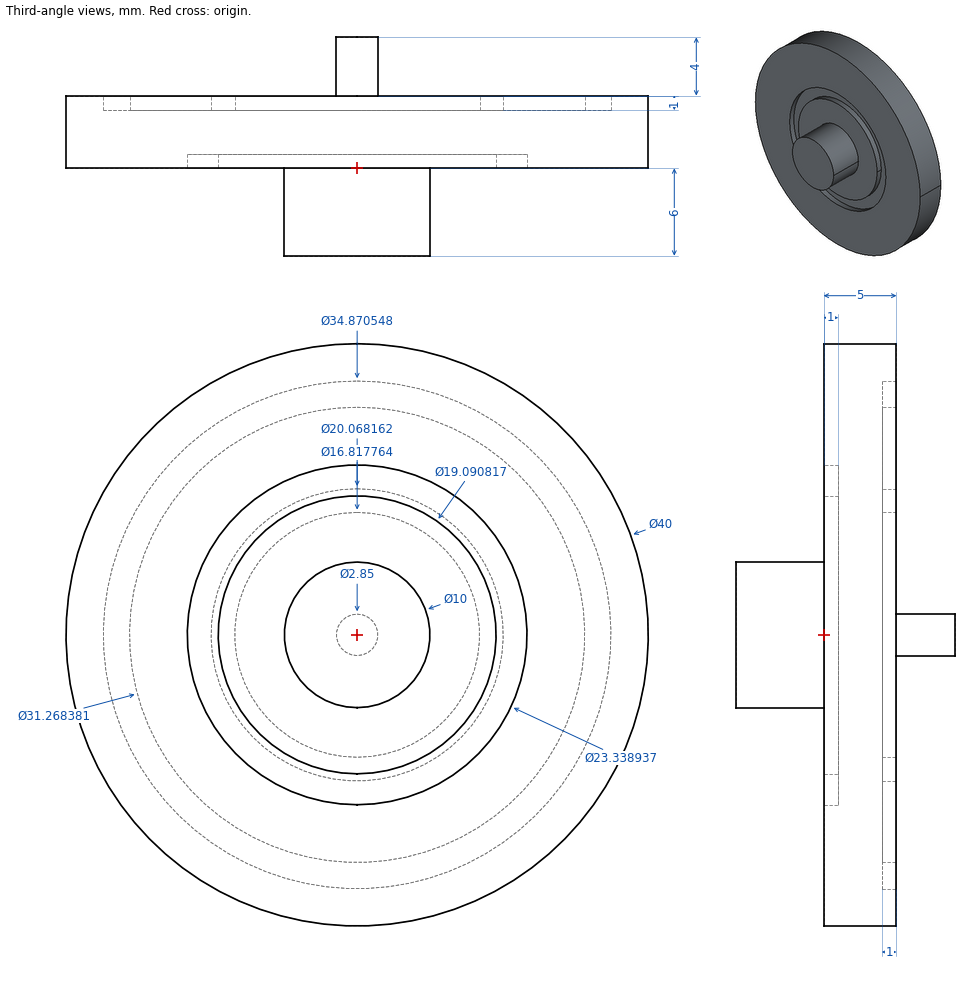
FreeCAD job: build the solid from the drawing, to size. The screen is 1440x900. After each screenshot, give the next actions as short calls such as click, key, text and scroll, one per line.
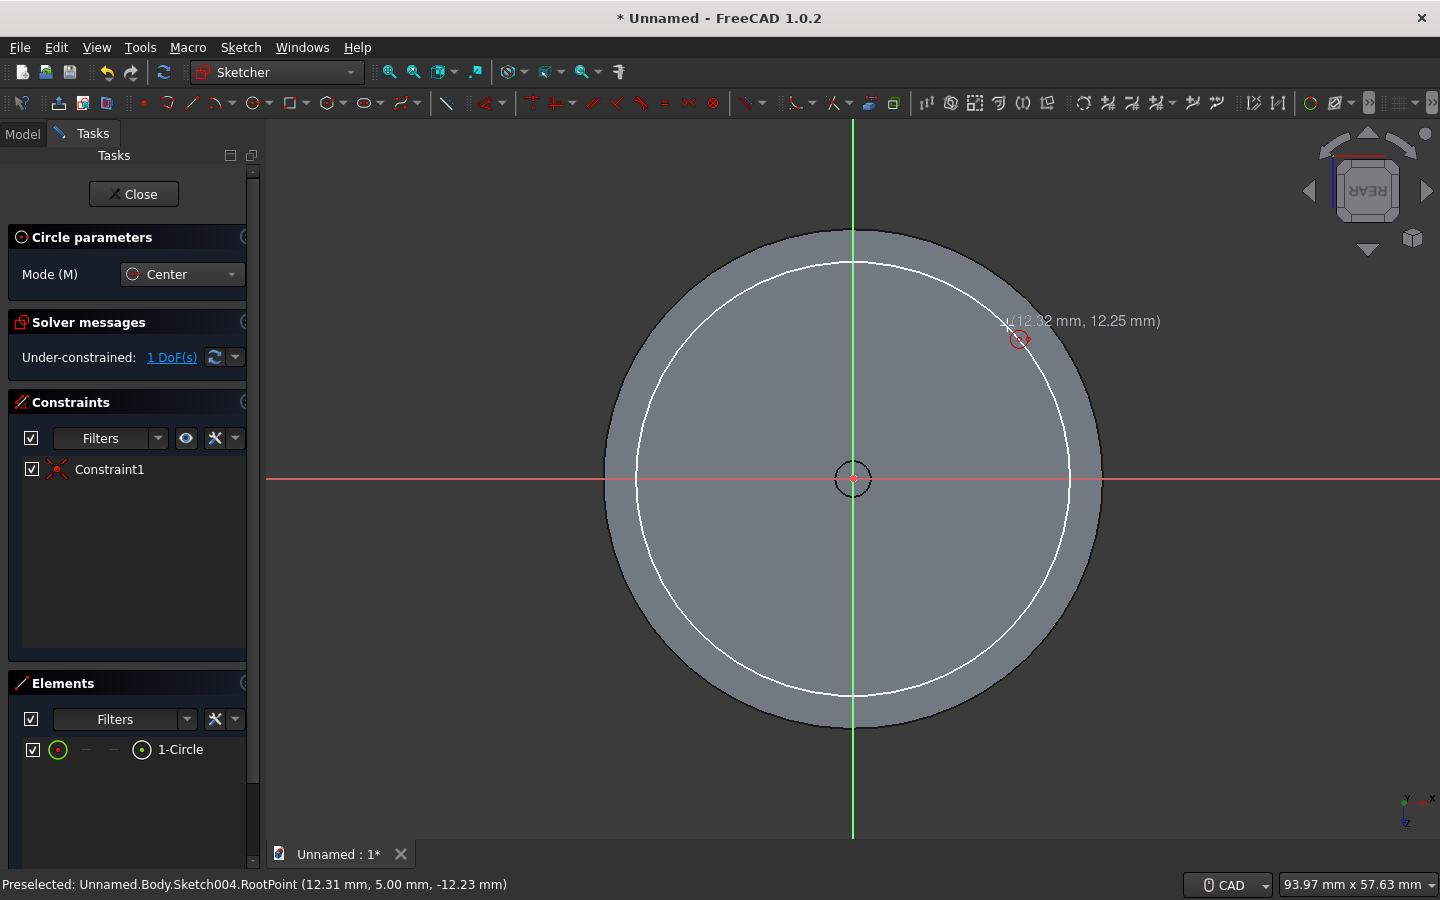
click(853, 479)
click(991, 341)
key(Escape)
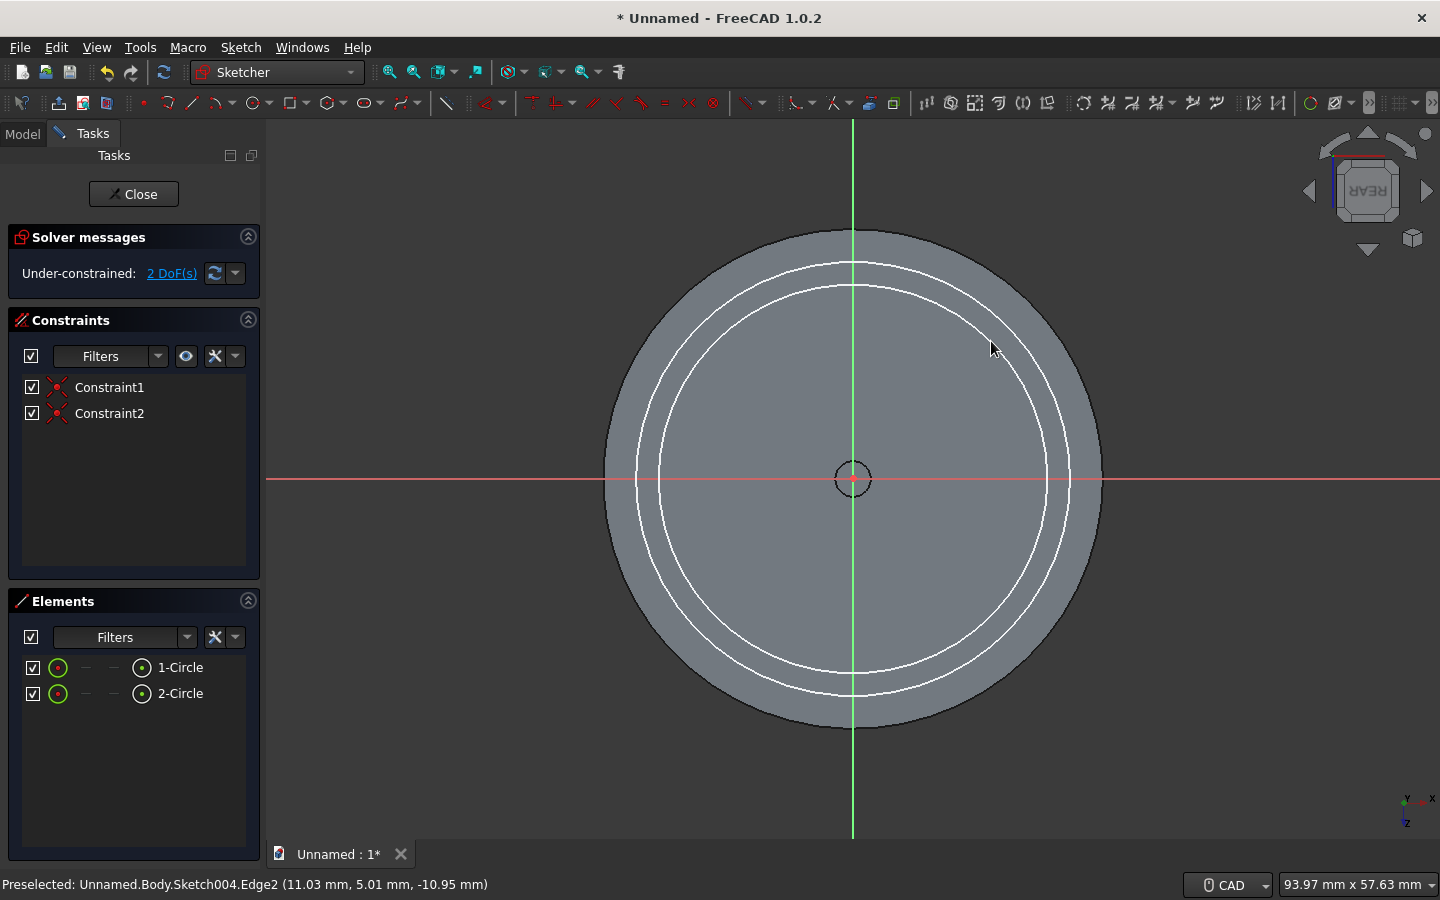
click(486, 104)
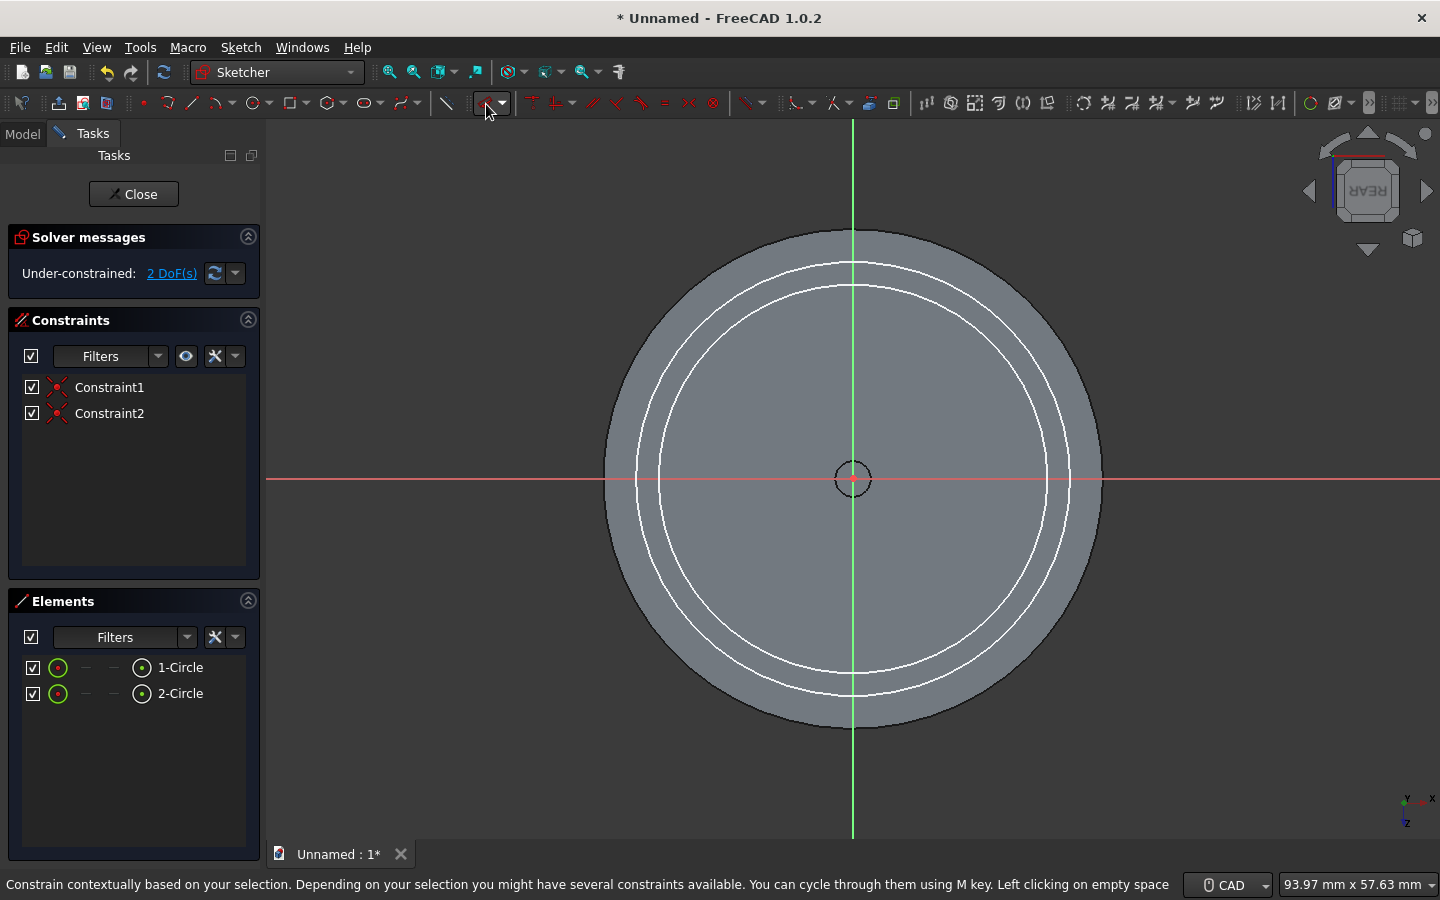
click(1006, 325)
click(1029, 302)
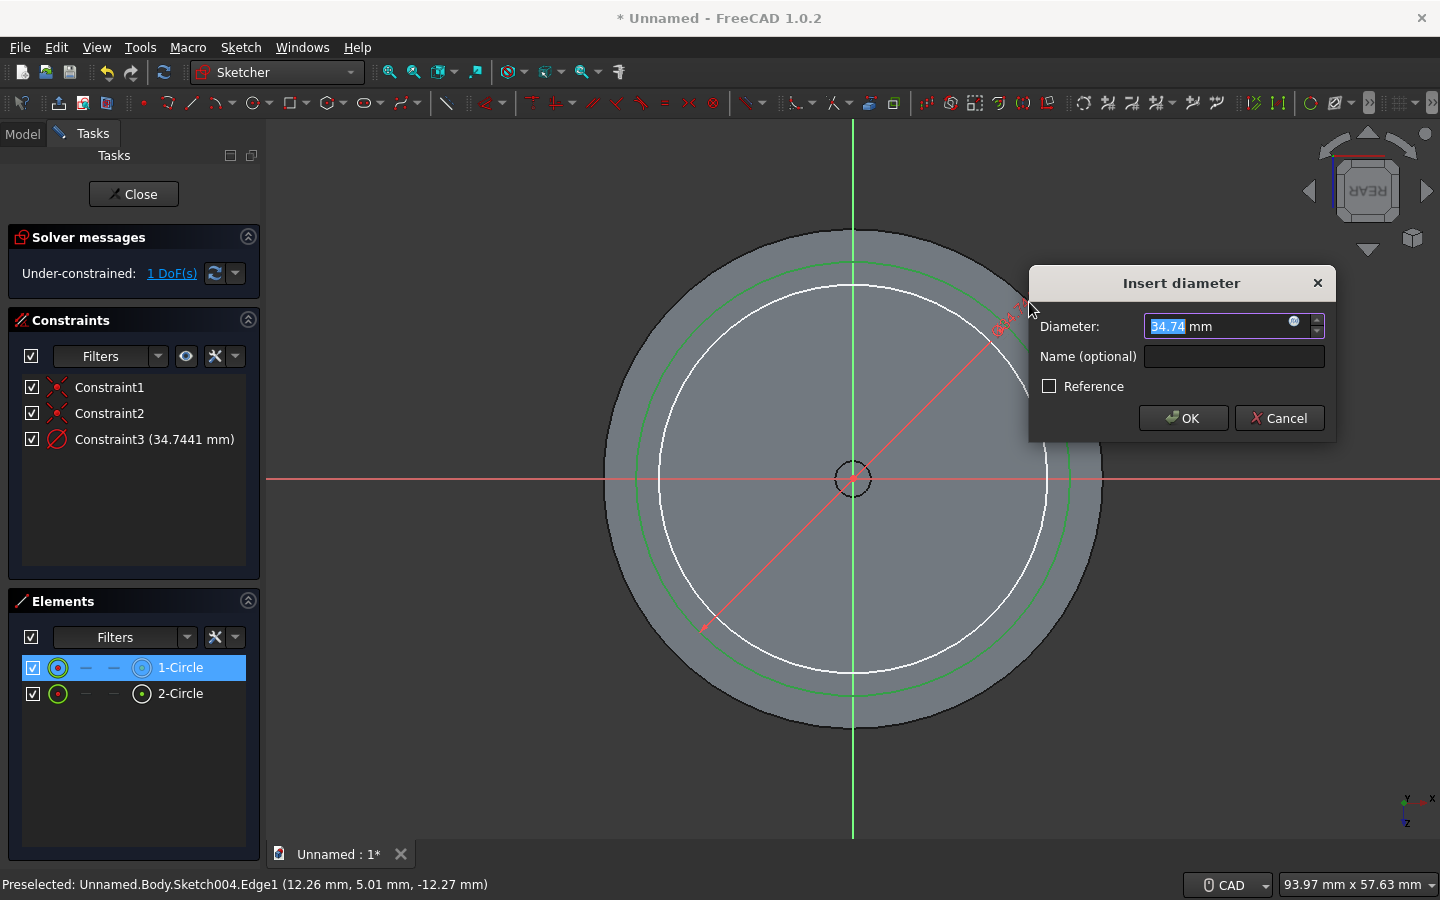
text(34.870548)
key(Return)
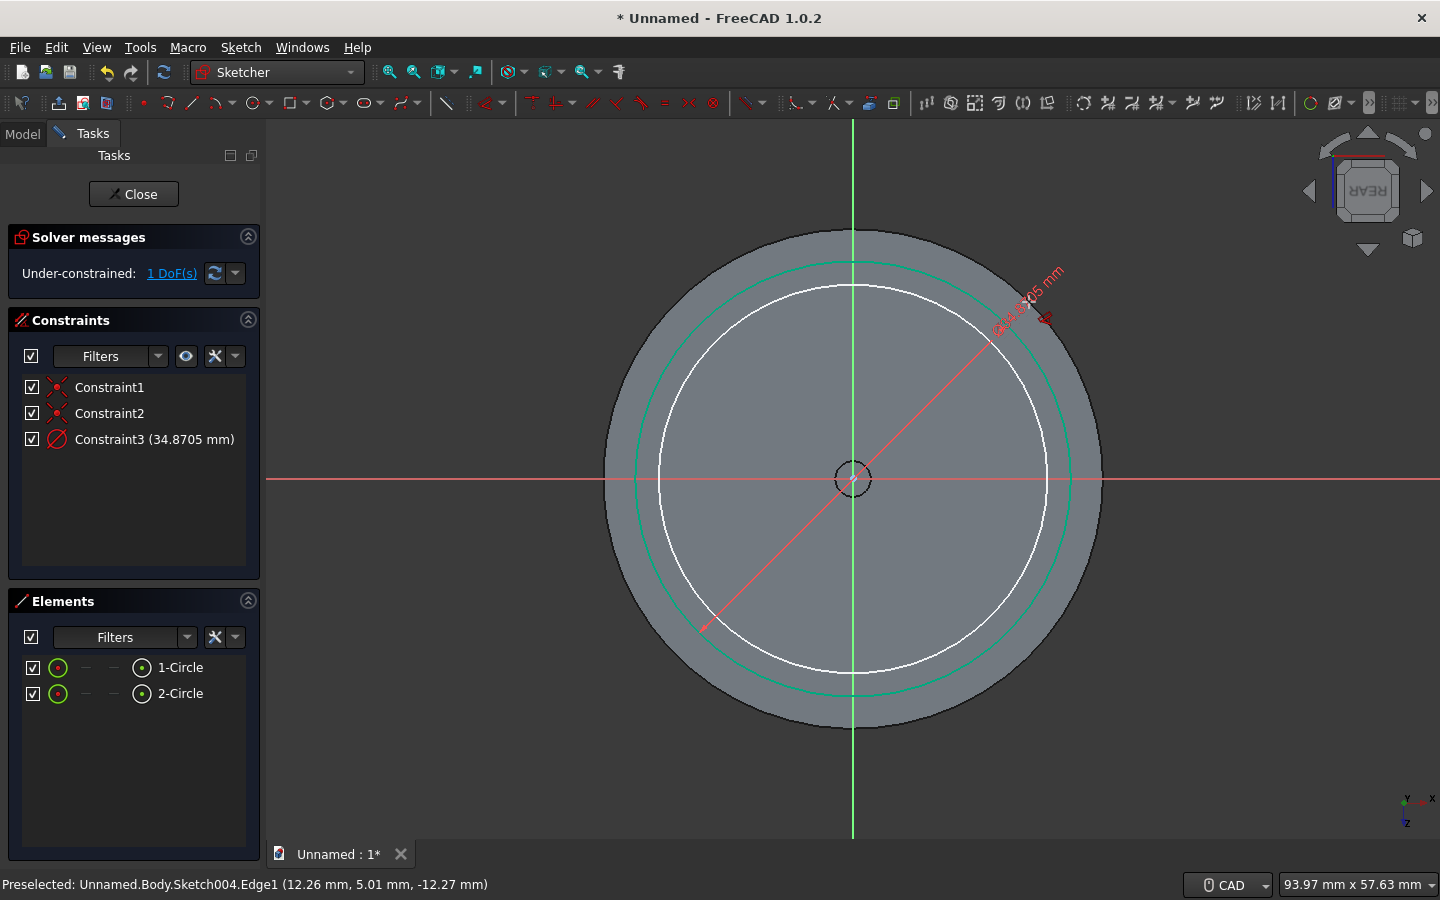
click(990, 341)
click(1092, 408)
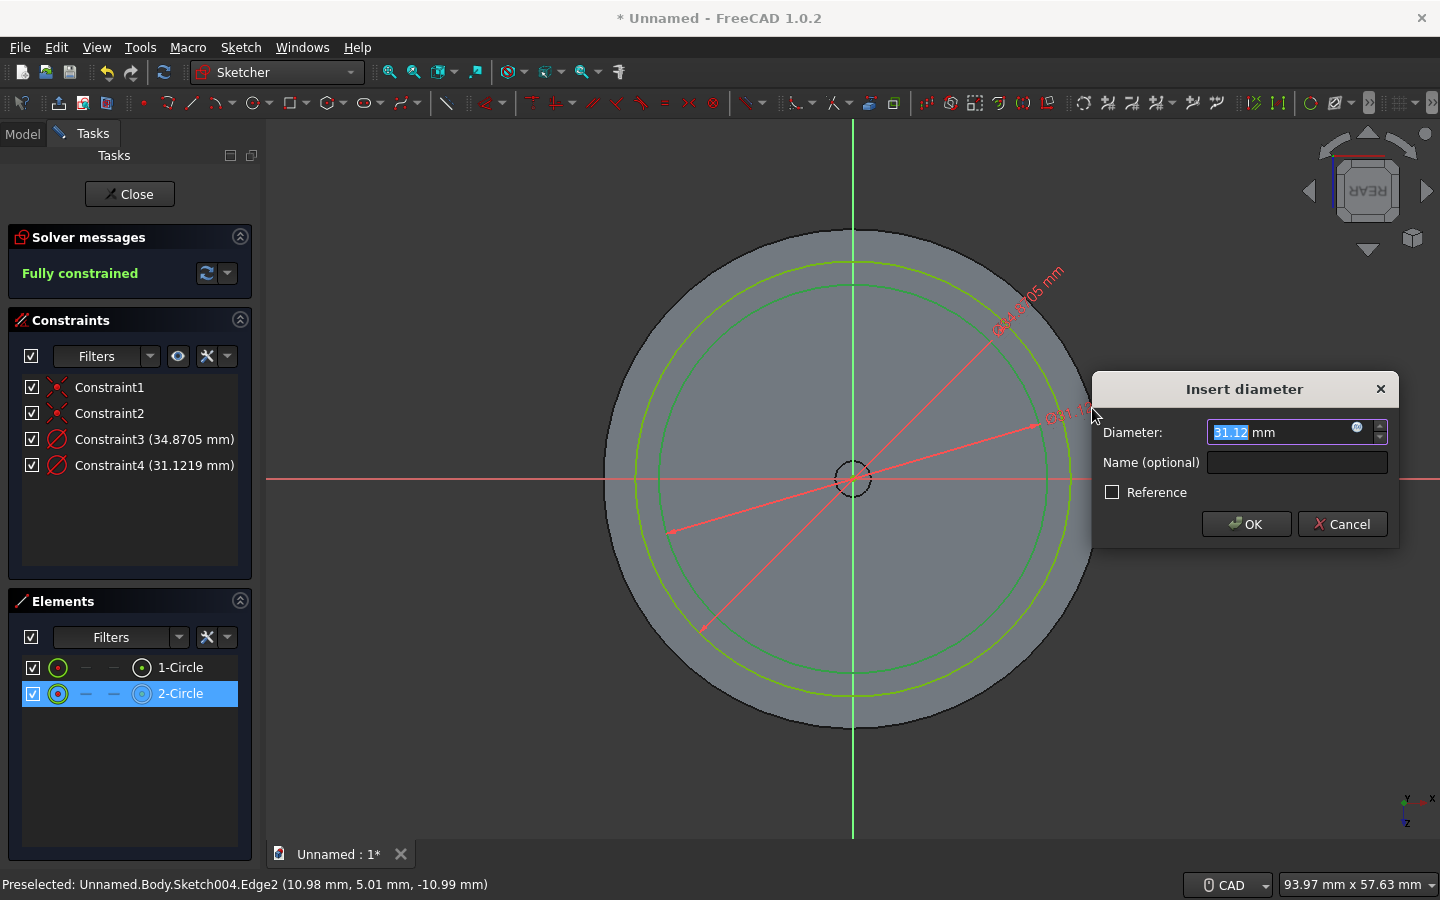
text(31.268381)
key(Return)
key(Escape)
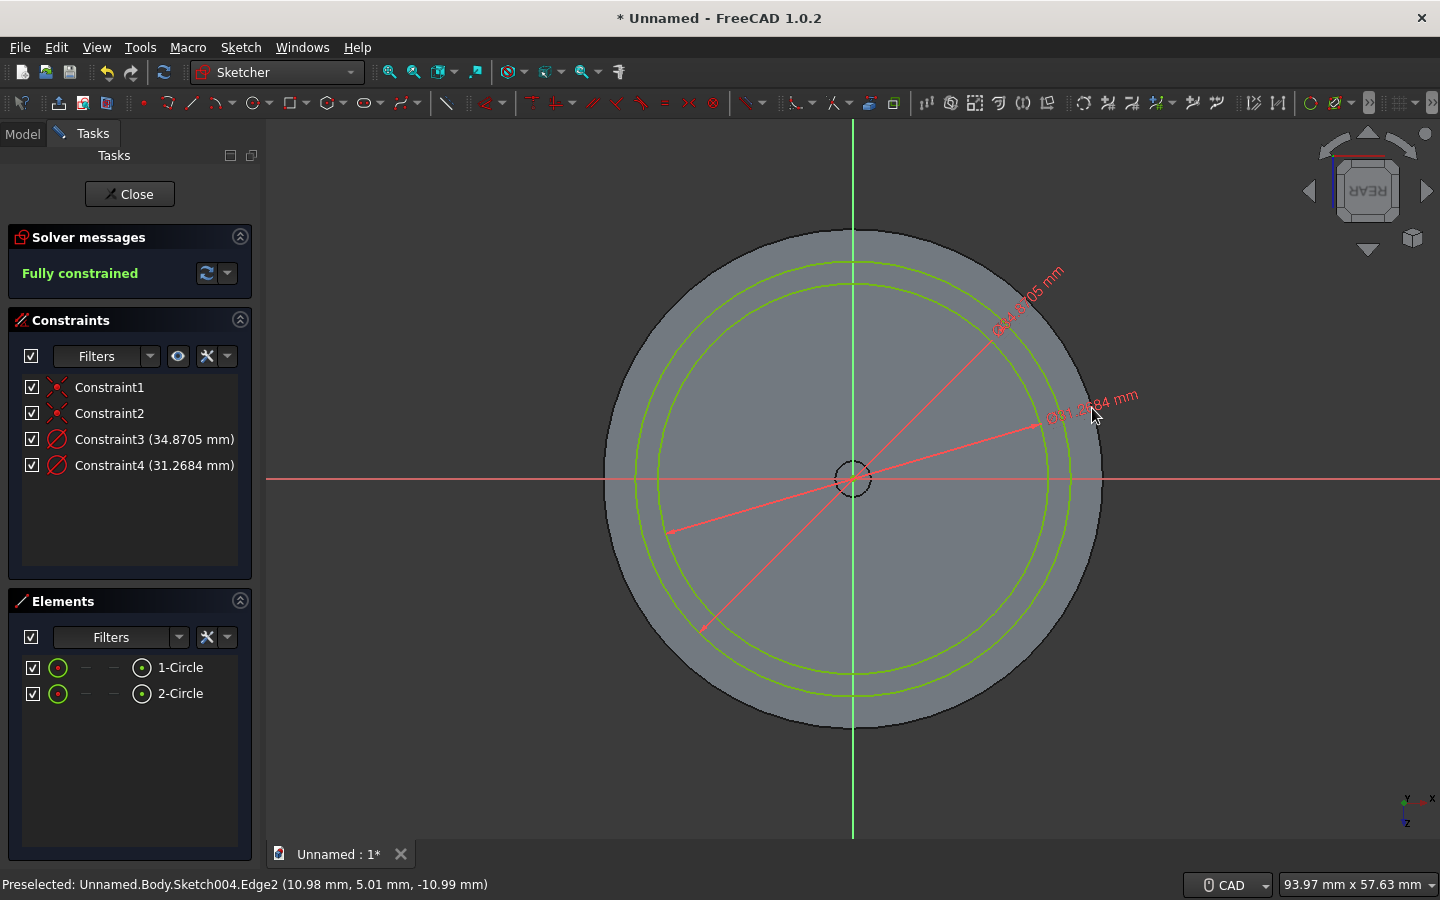
click(130, 194)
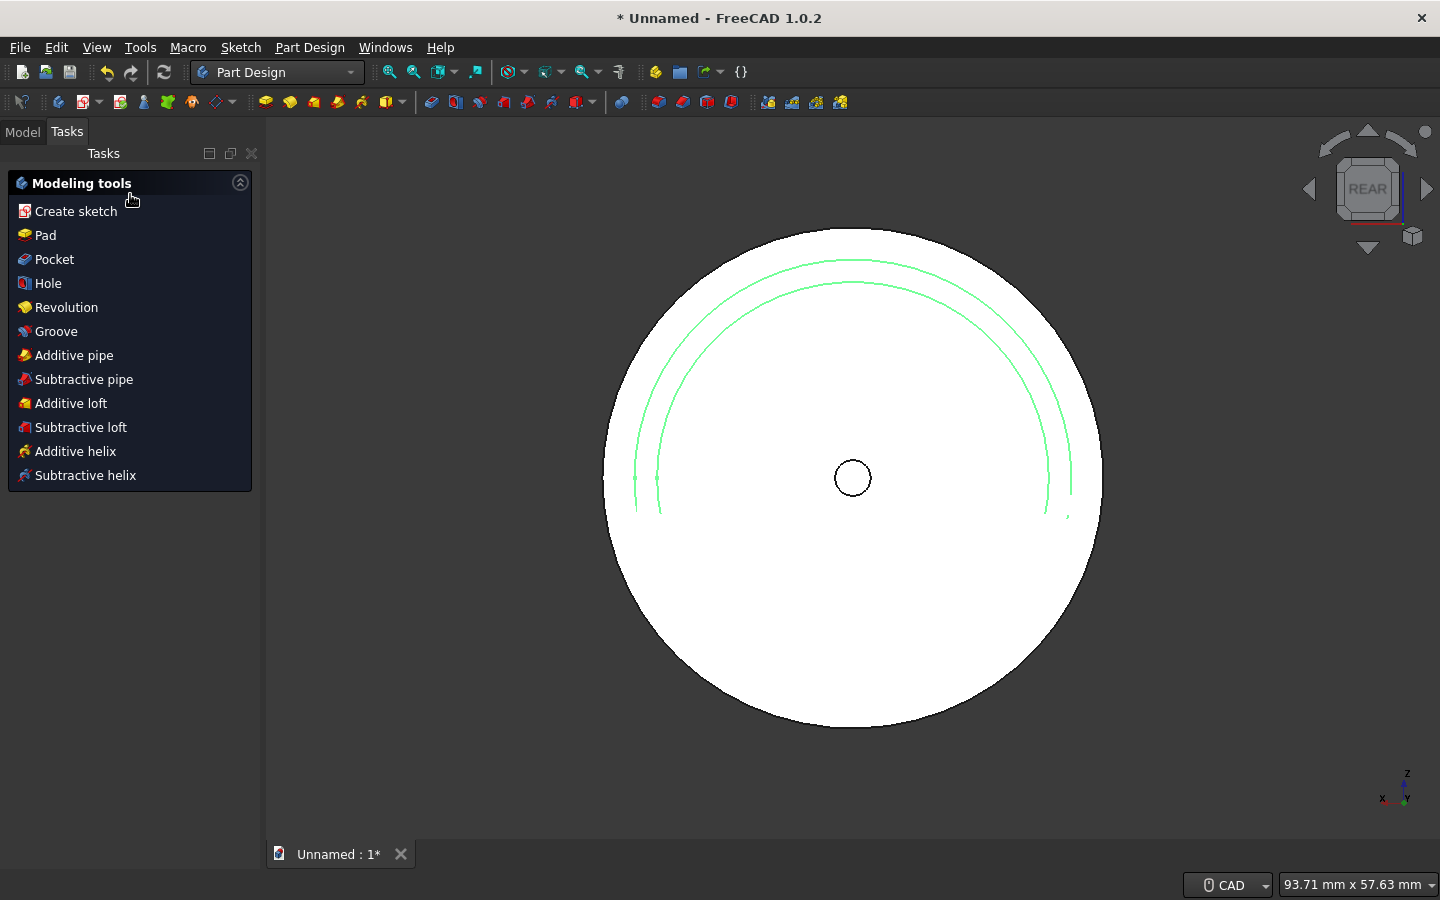
click(432, 102)